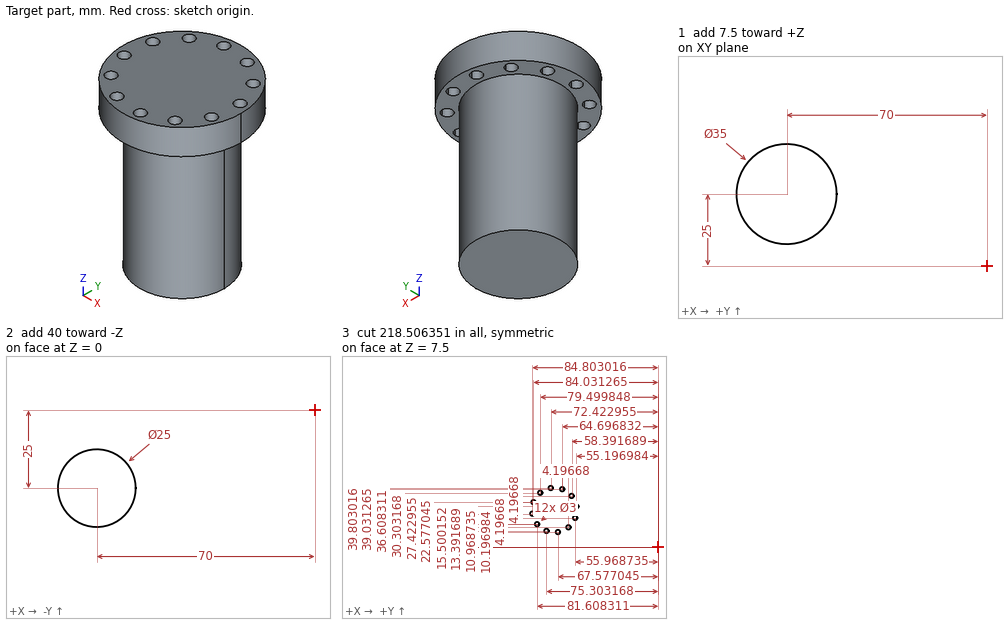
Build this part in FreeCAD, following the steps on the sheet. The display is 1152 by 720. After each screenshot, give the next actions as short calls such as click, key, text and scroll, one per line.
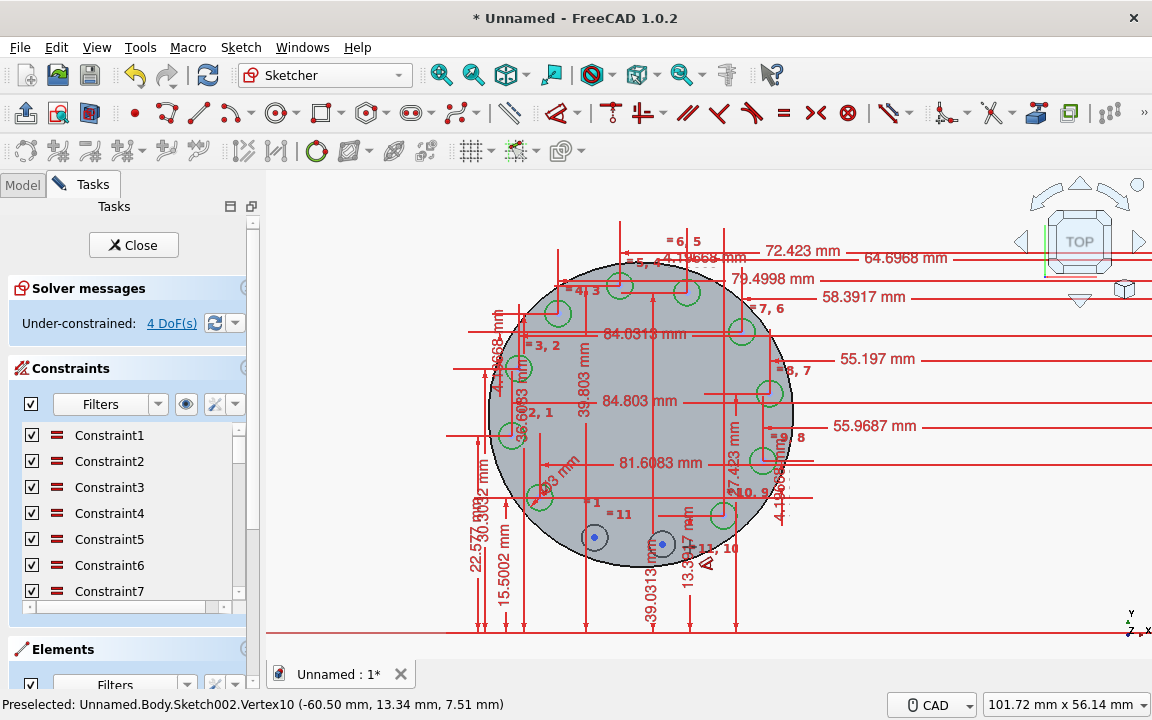
click(662, 544)
click(825, 510)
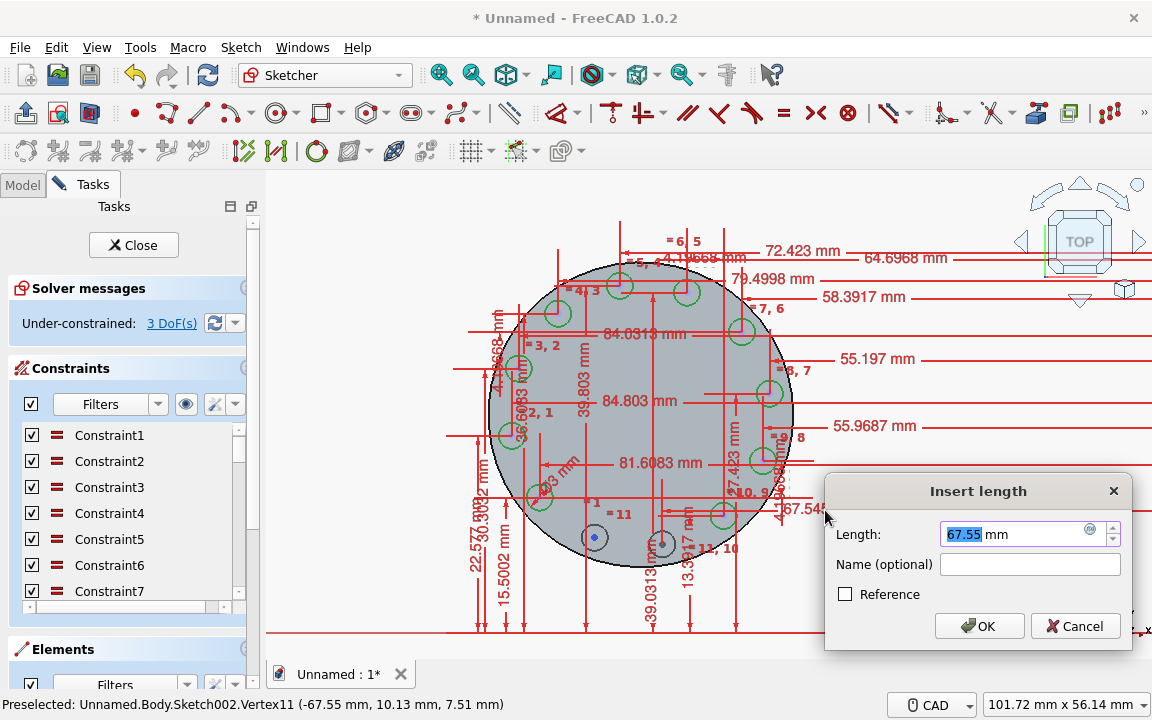
text(67.577045)
key(Return)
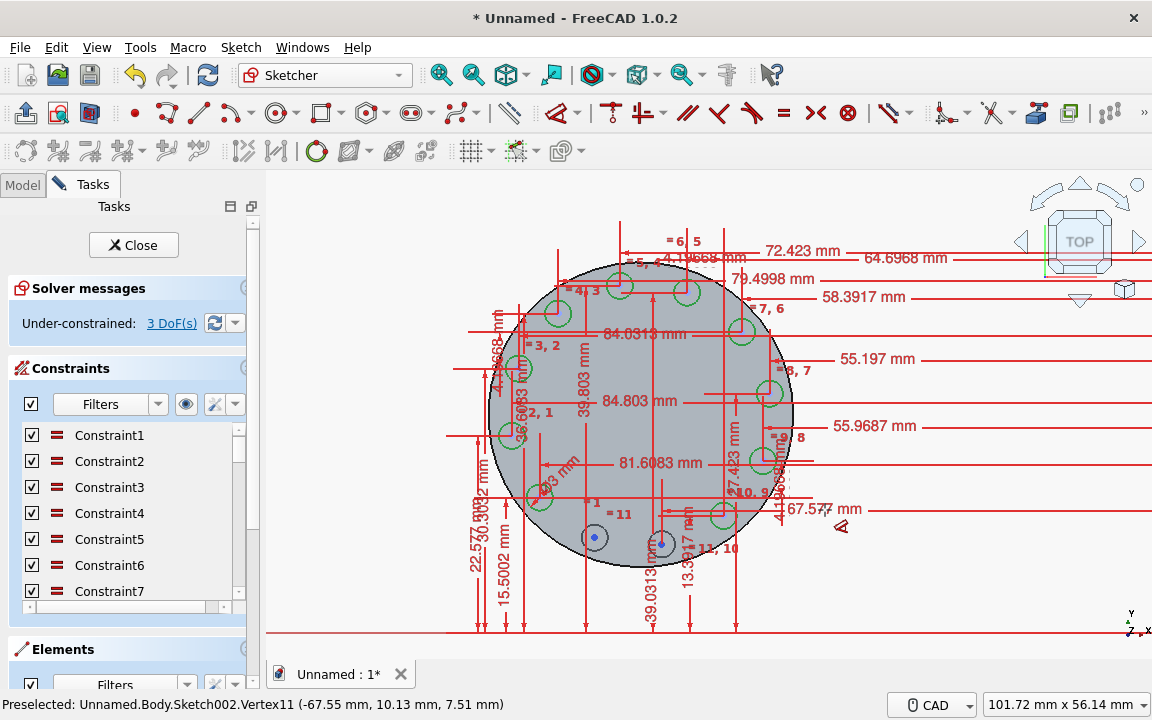
click(662, 544)
click(628, 608)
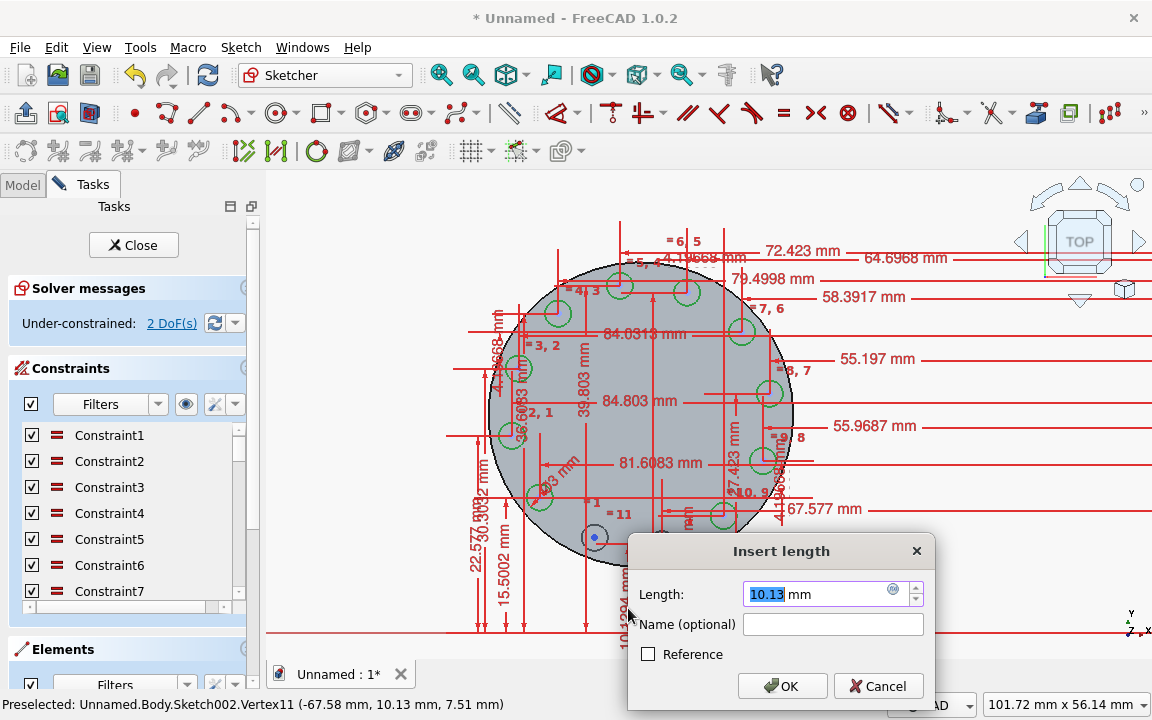
text(10.196984)
key(Return)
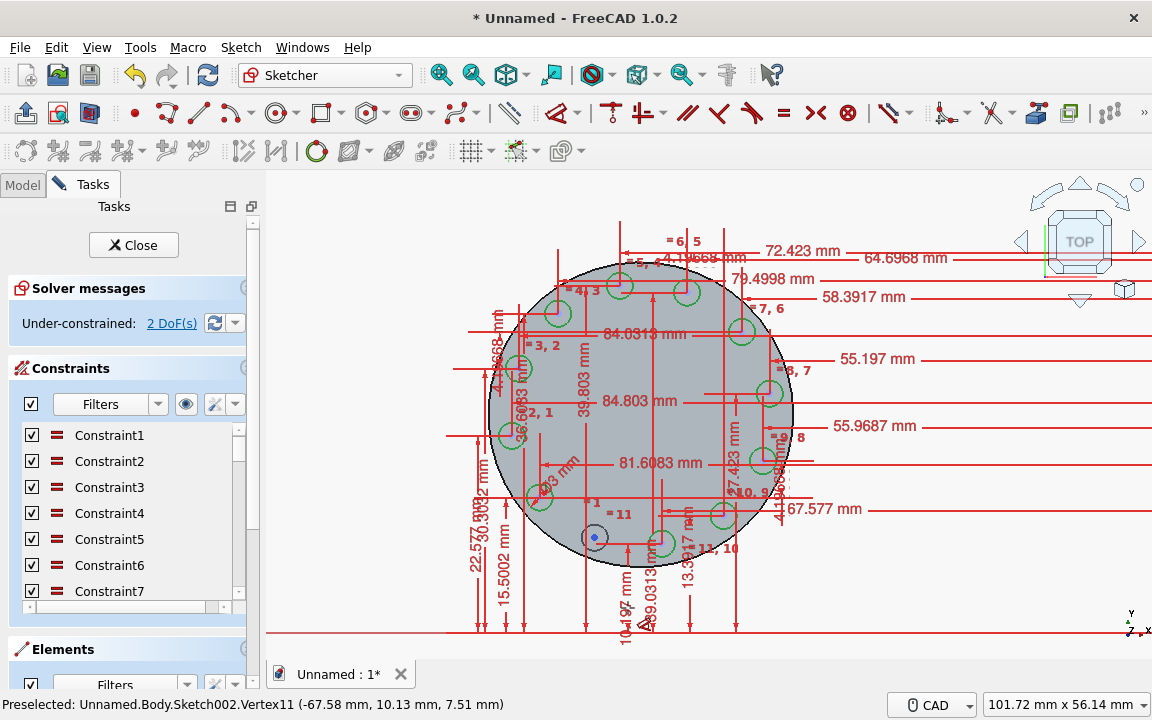
click(595, 538)
click(654, 504)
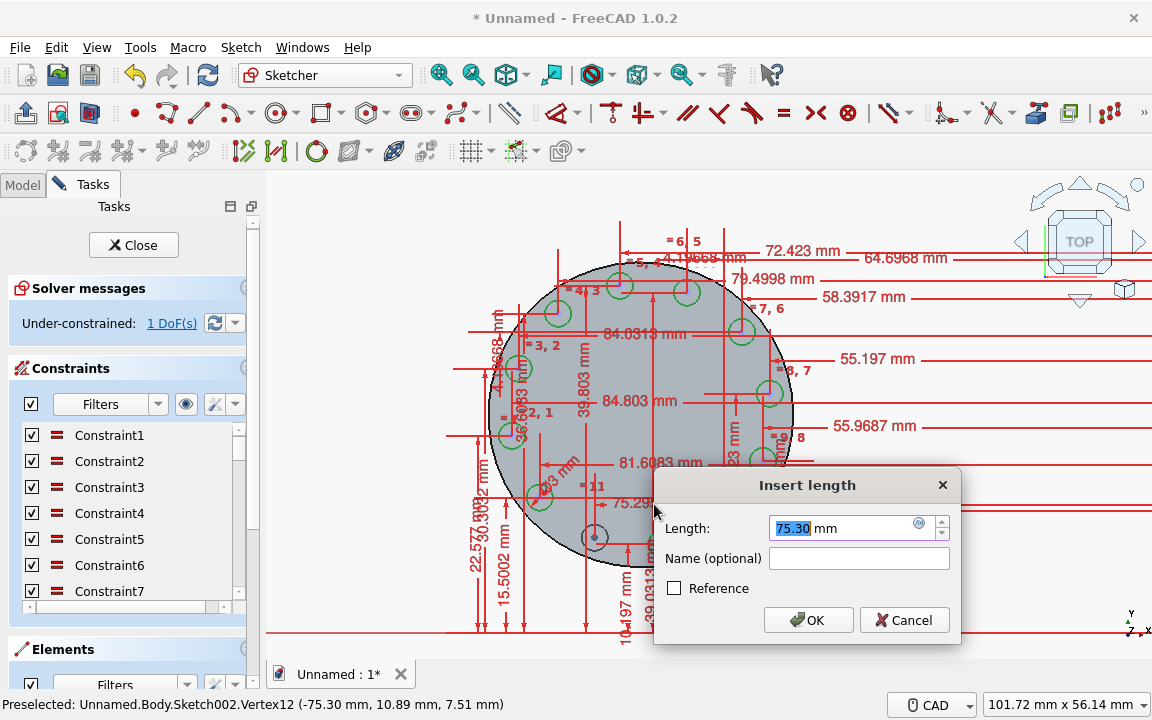
text(75.303168)
key(Return)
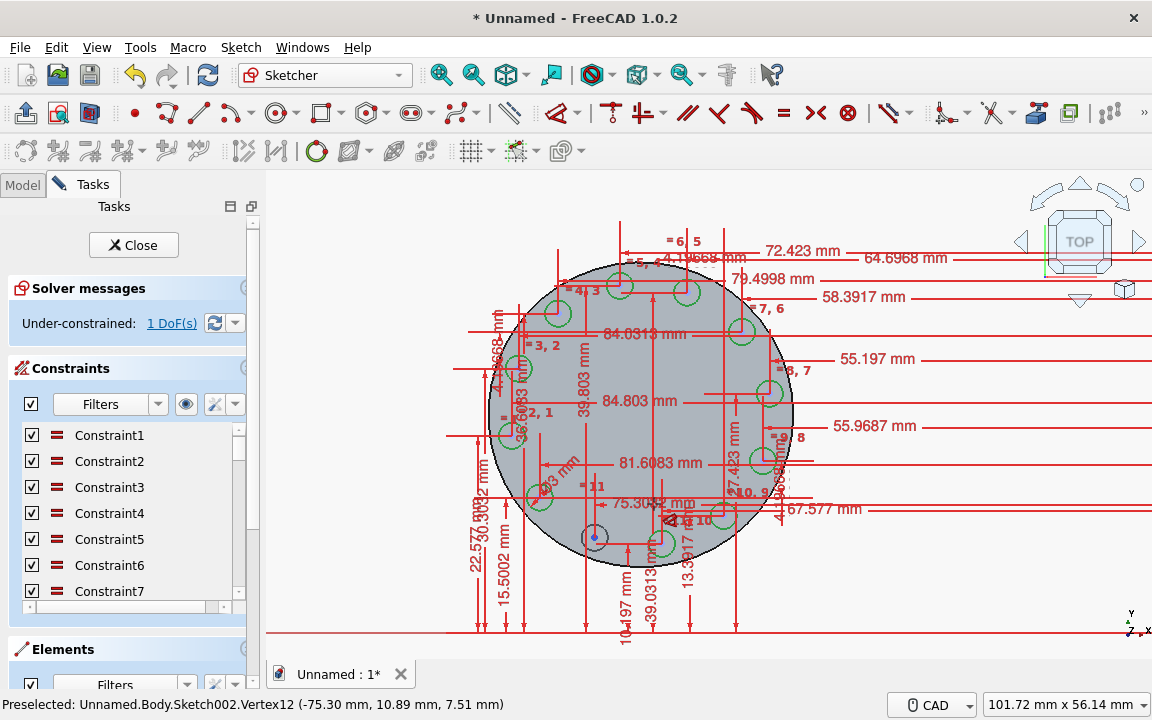
click(595, 538)
click(537, 606)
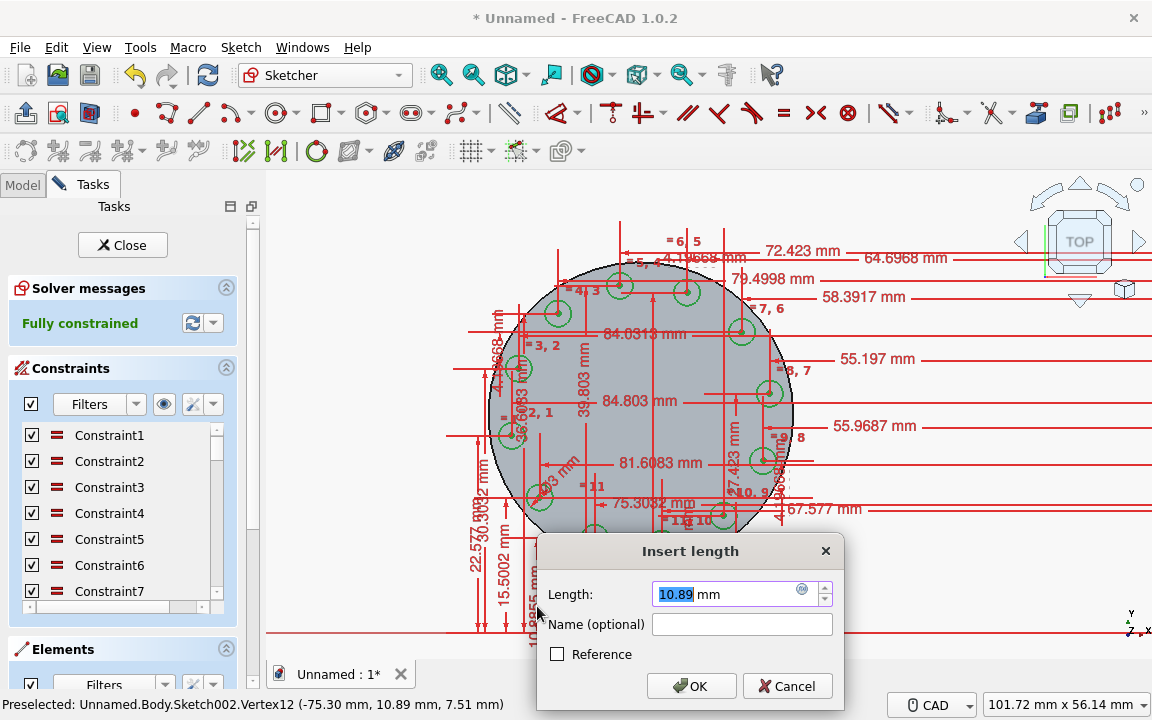
text(10.968735)
key(Return)
key(Escape)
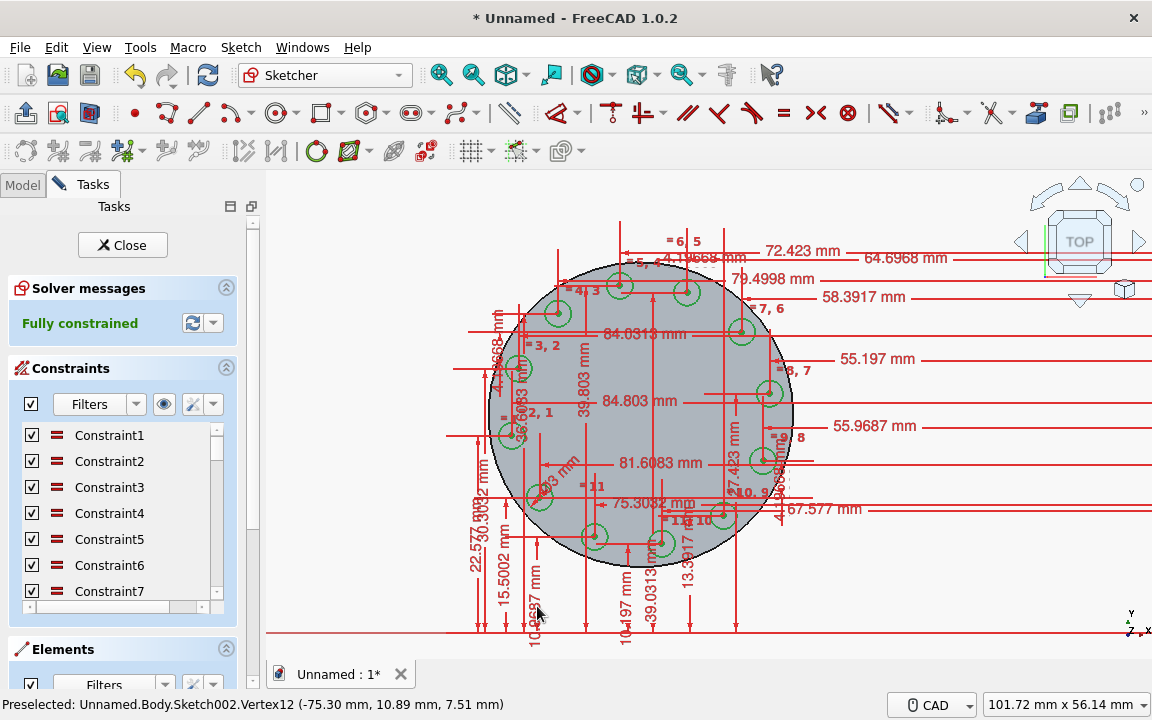
click(123, 245)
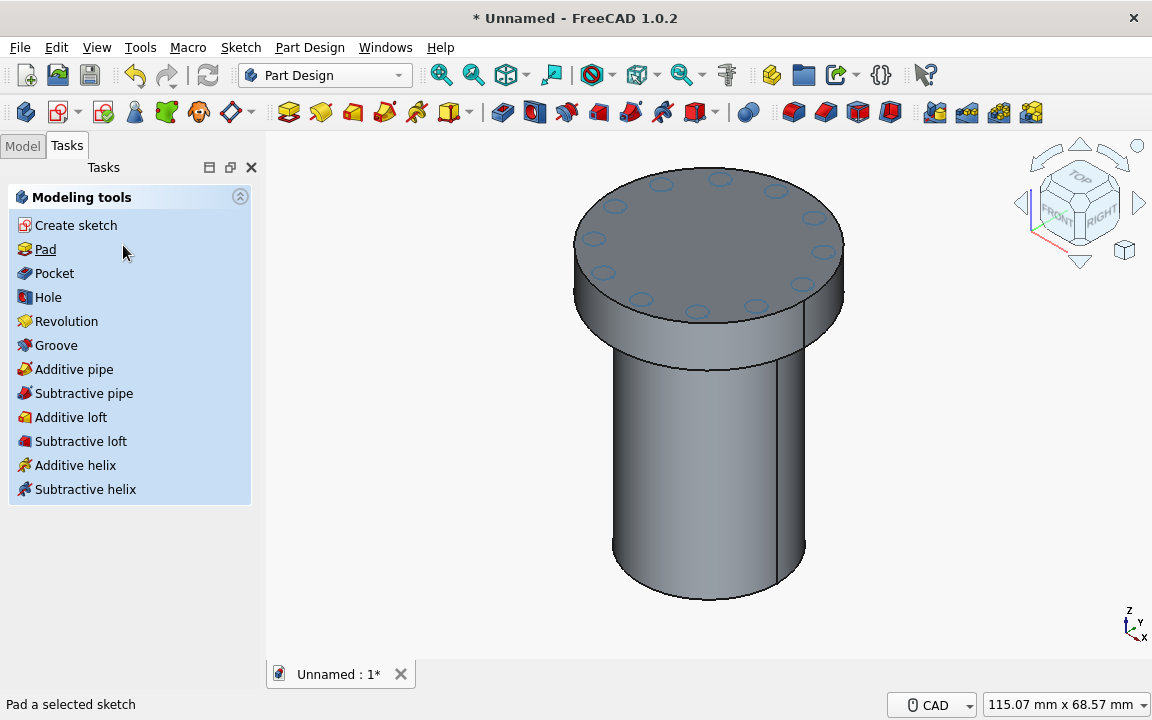
click(504, 112)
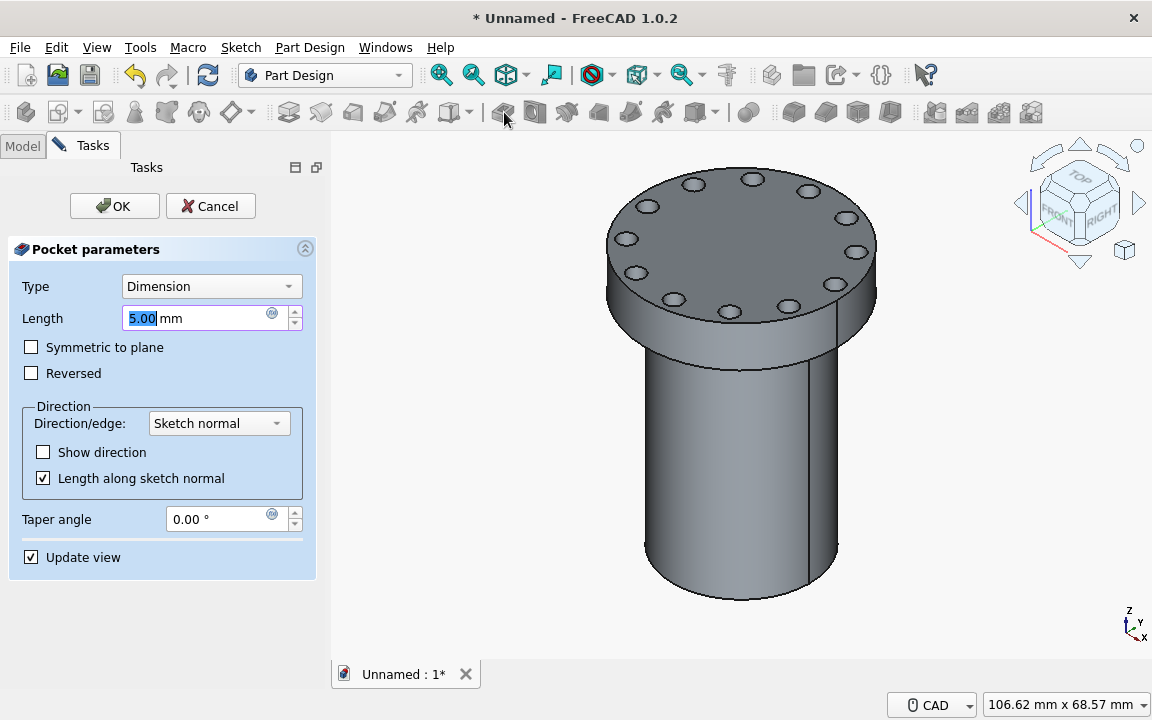
text(218.506351)
key(Tab)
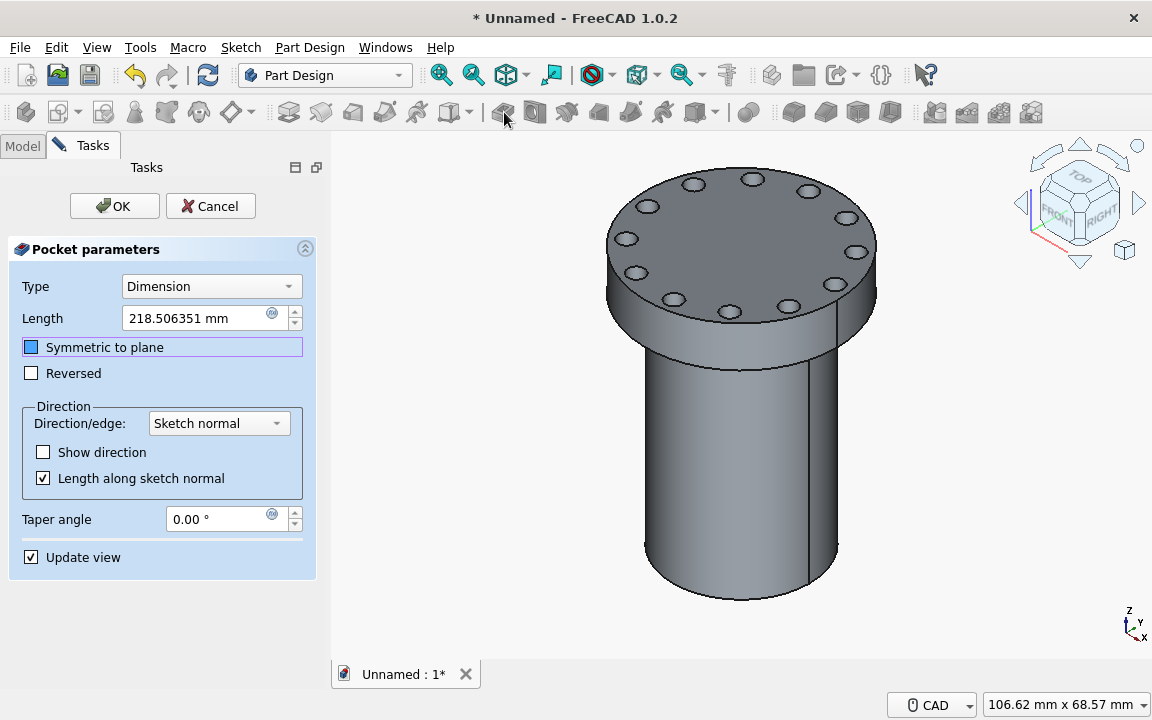
click(30, 347)